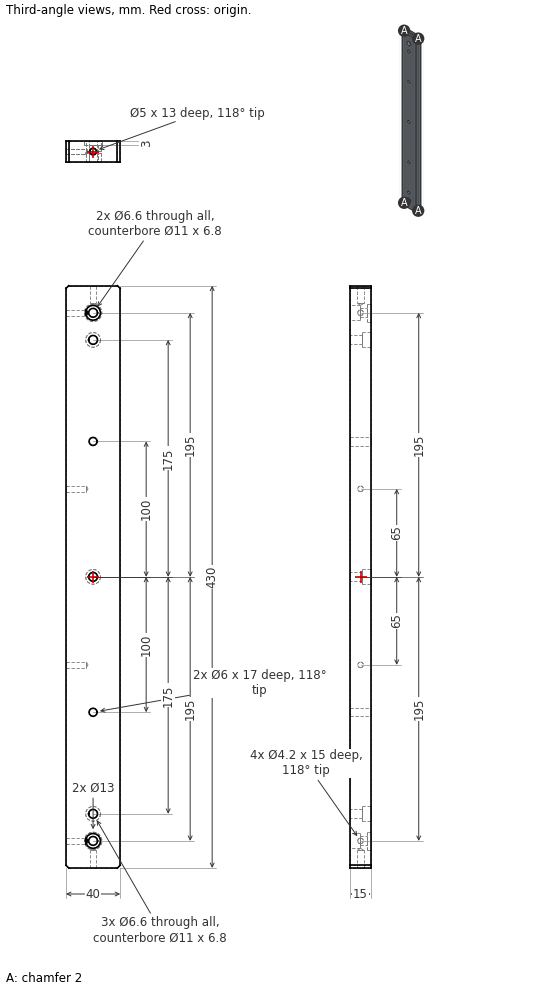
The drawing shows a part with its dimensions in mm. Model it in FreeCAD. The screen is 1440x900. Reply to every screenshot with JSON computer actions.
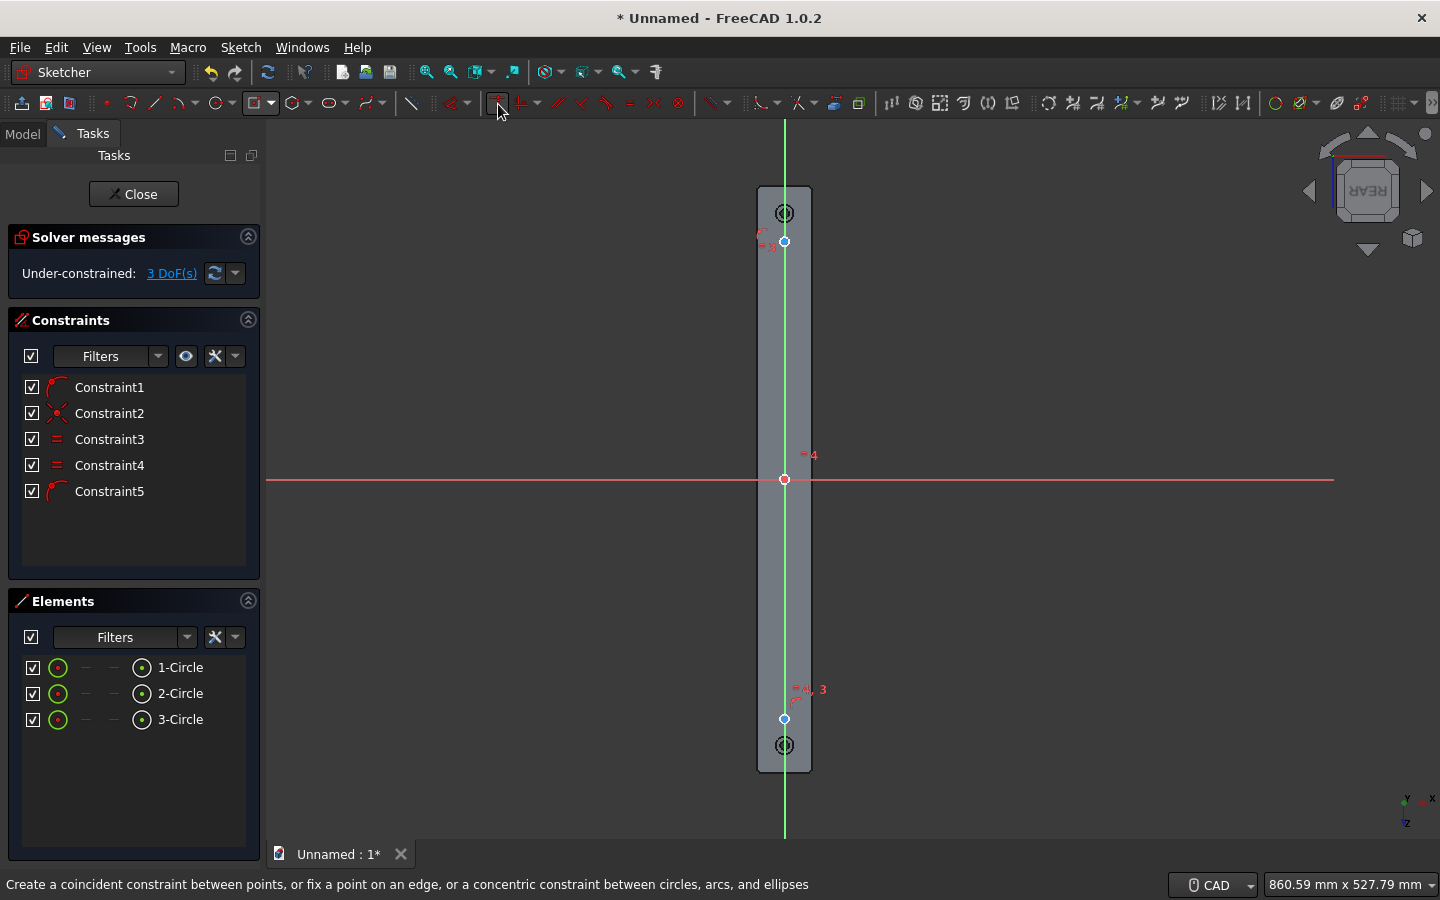
{"action": "key", "text": "d"}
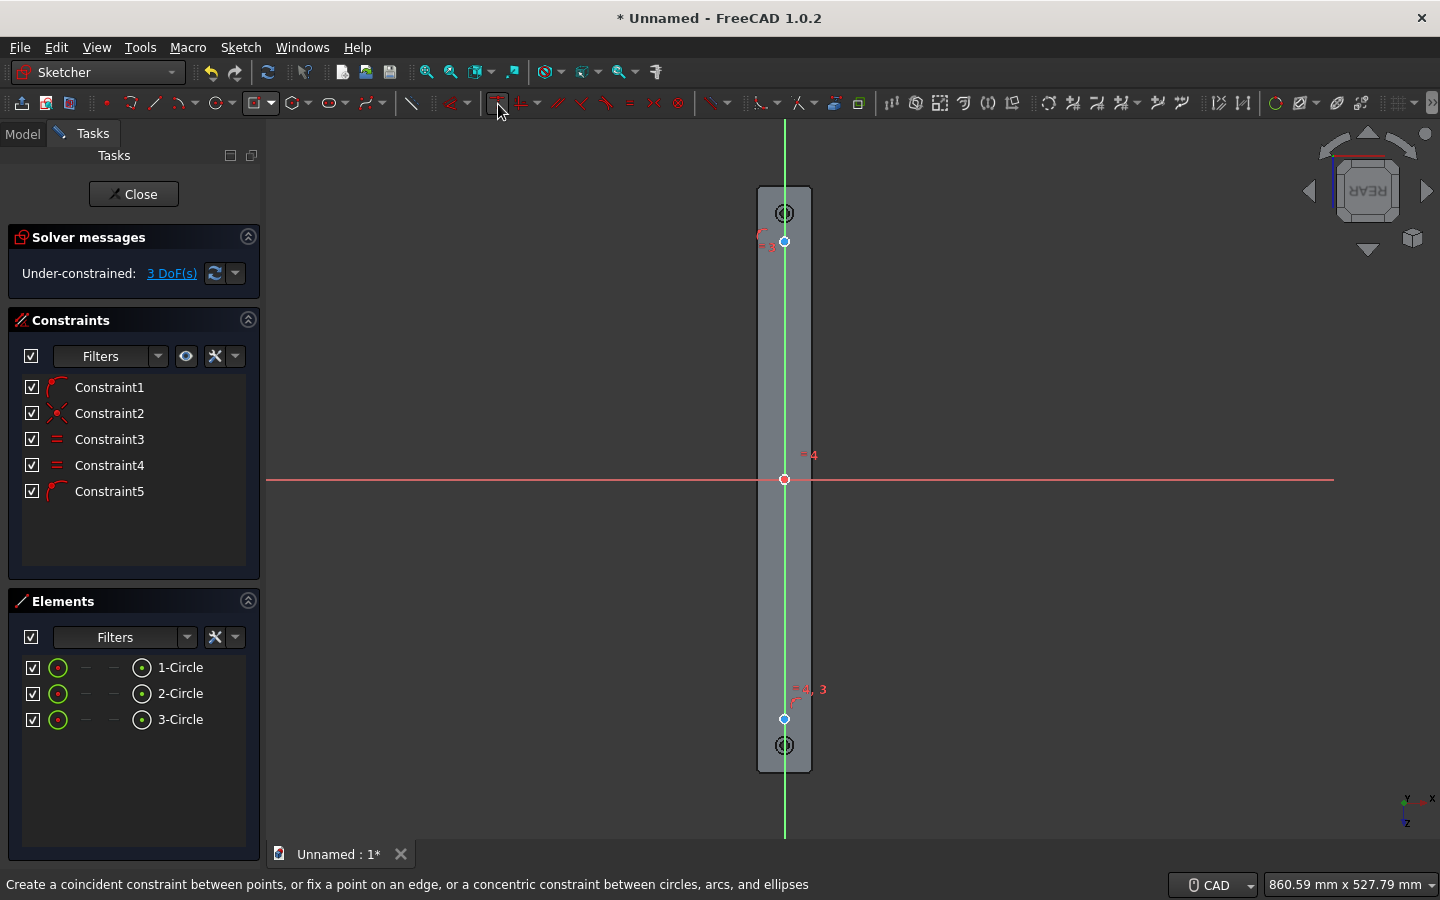
{"action": "scroll", "coordinate": [785, 237], "scroll_direction": "up", "scroll_amount": 8}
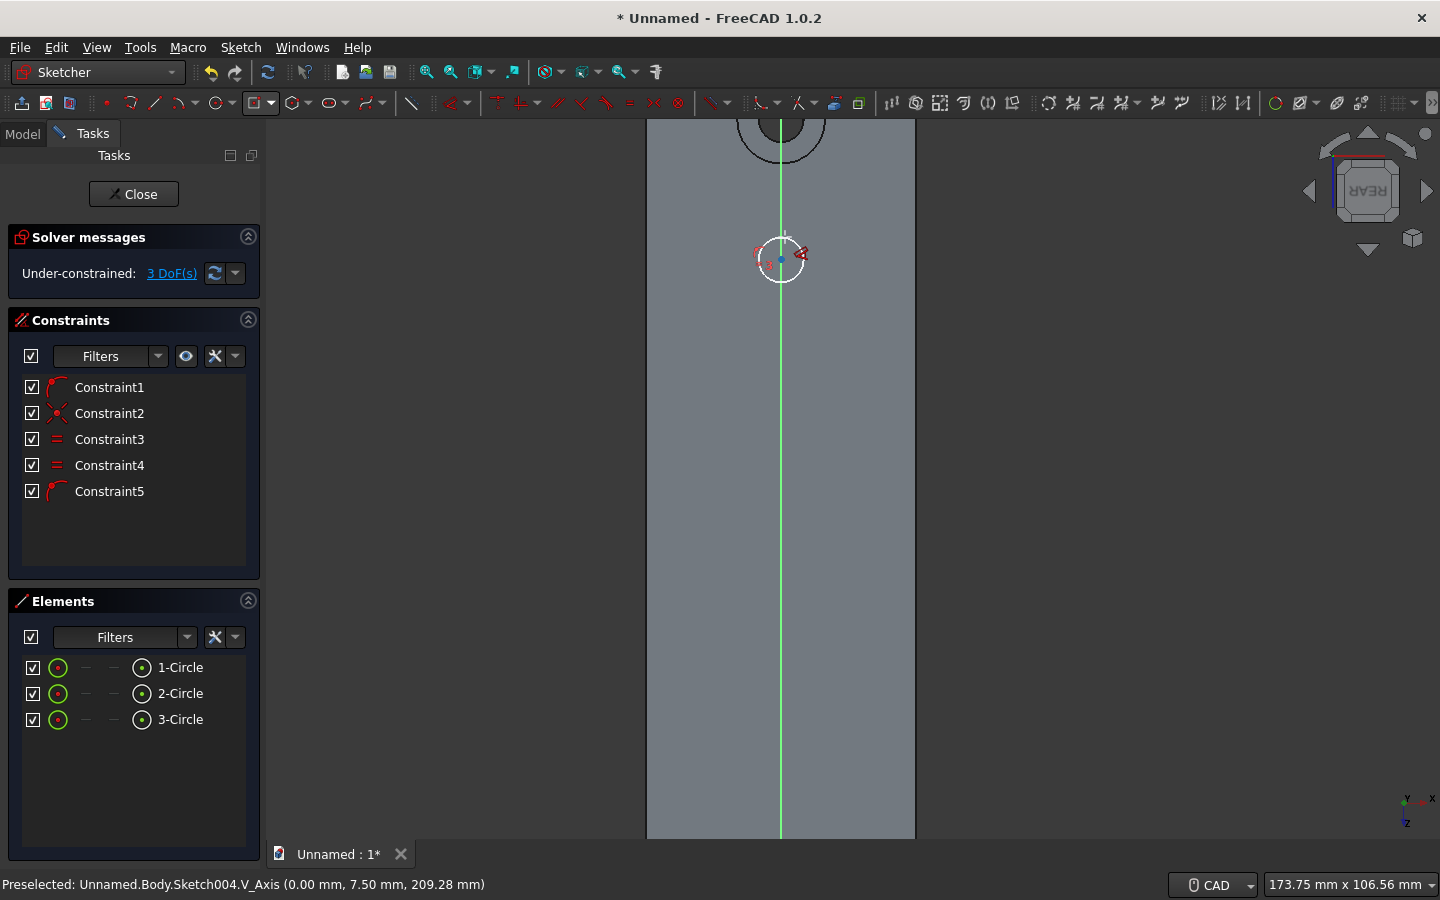
{"action": "left_click", "coordinate": [782, 238]}
{"action": "left_click", "coordinate": [809, 214]}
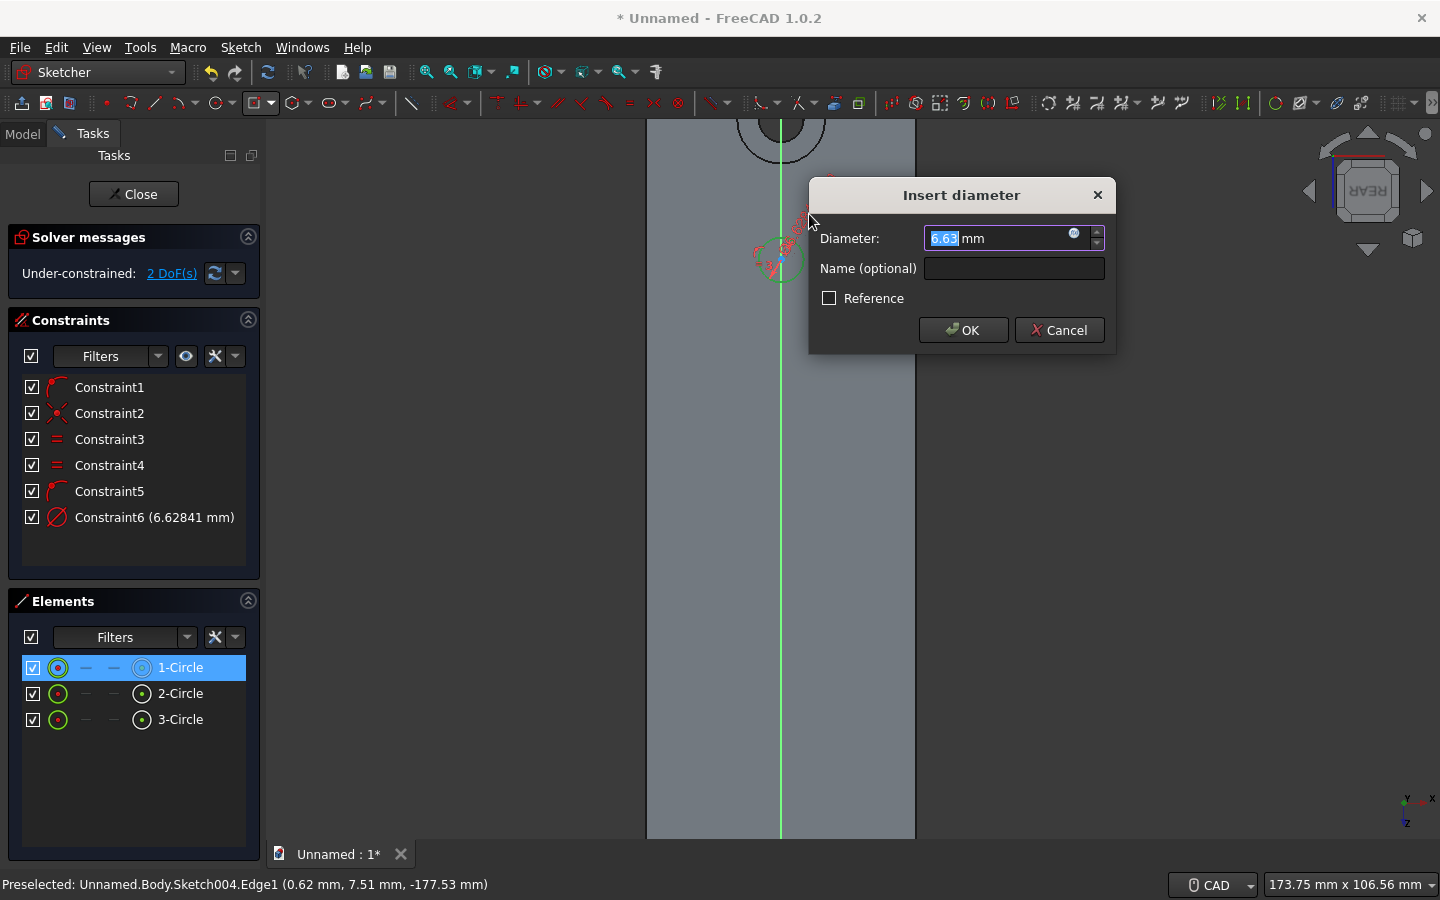
{"action": "type", "text": "6.6"}
{"action": "key", "text": "Return"}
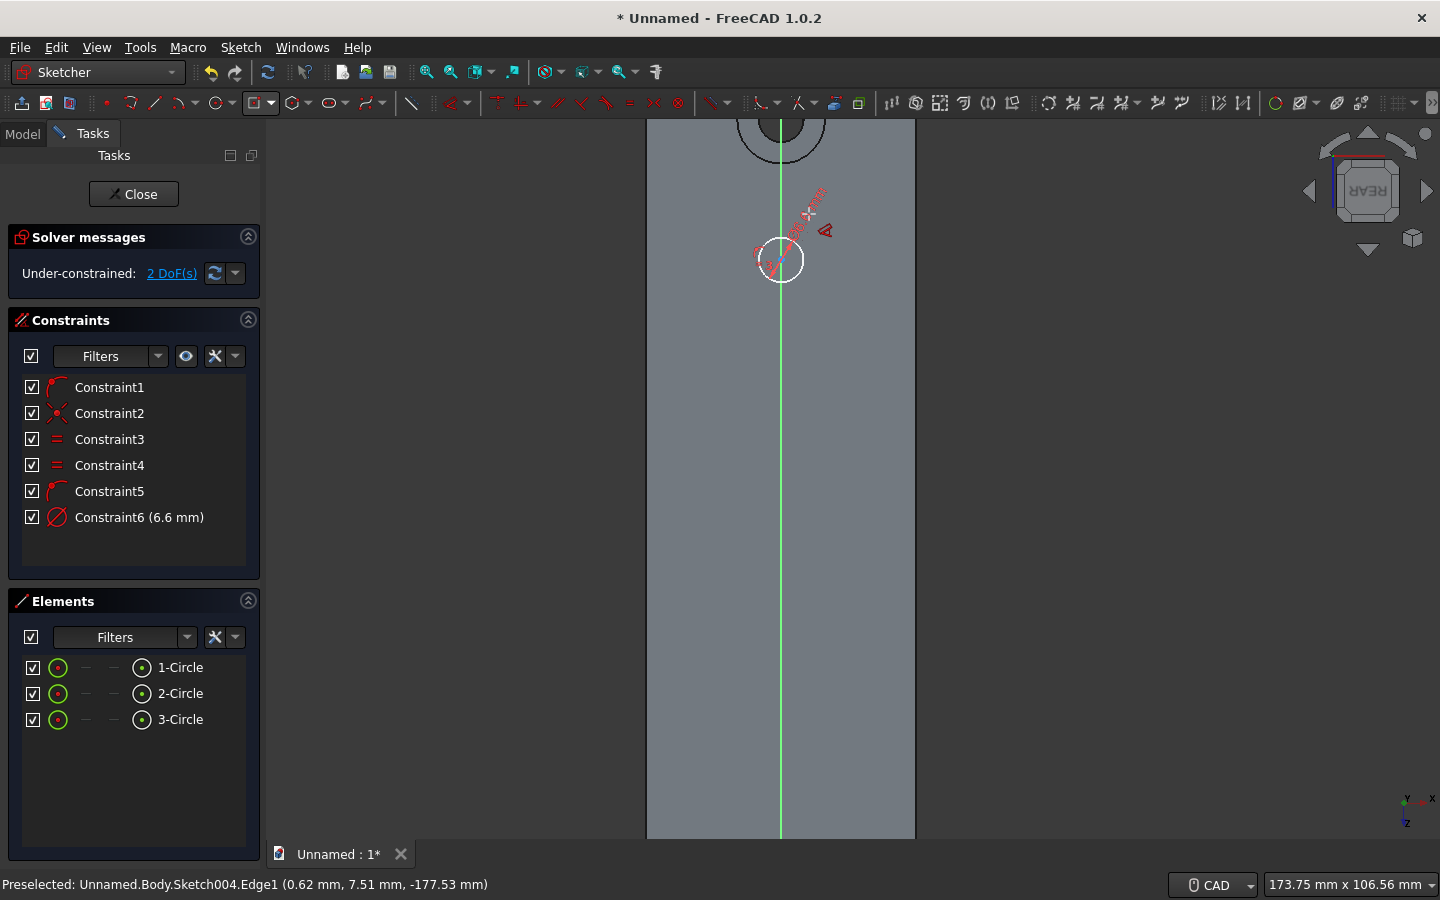
{"action": "scroll", "coordinate": [785, 237], "scroll_direction": "down", "scroll_amount": 8}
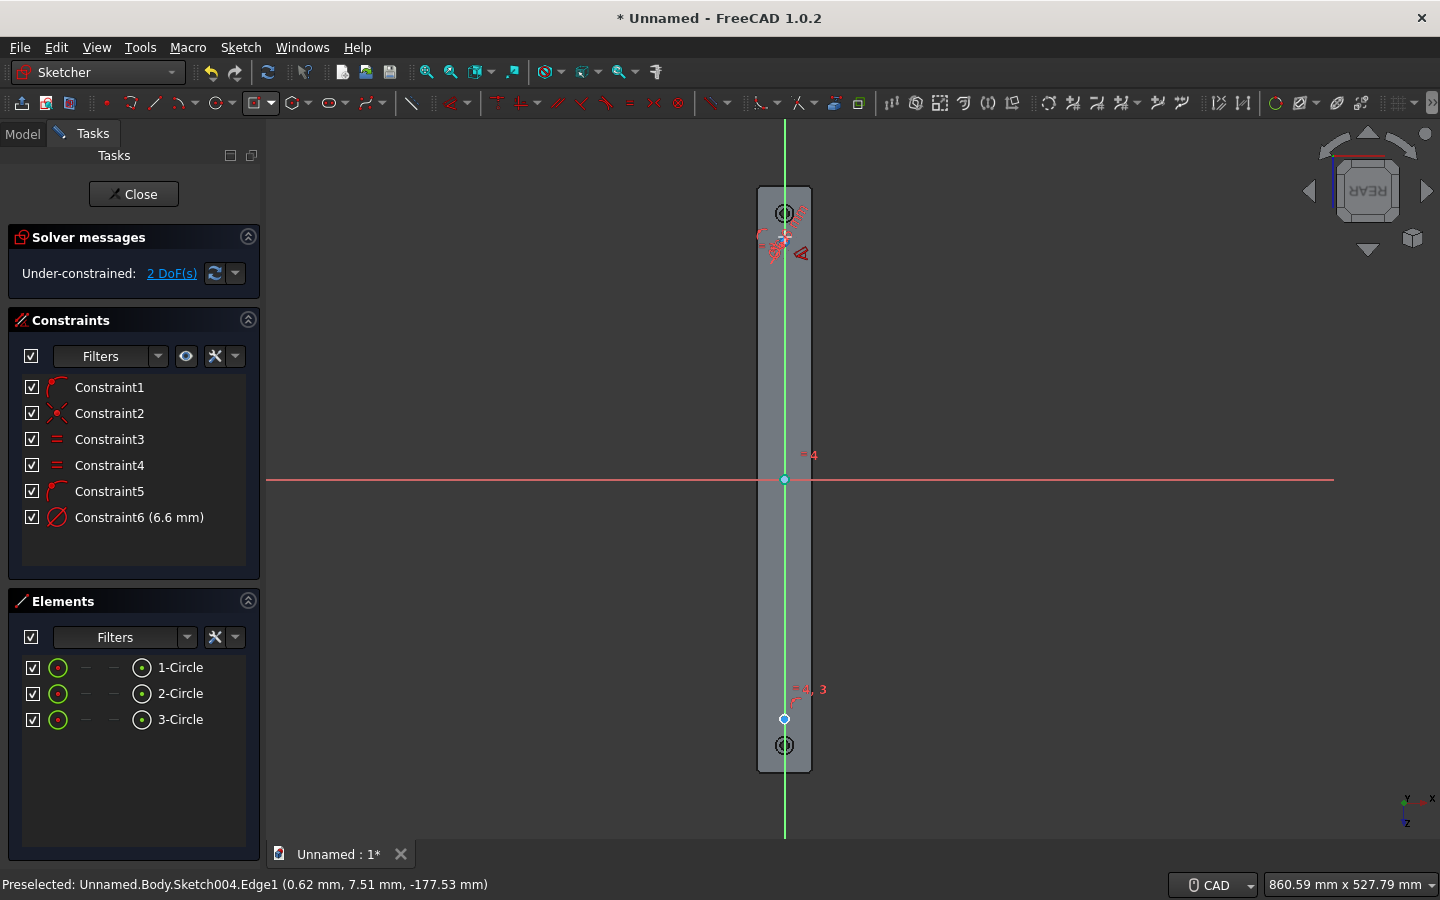
{"action": "left_click", "coordinate": [785, 242]}
{"action": "left_click", "coordinate": [819, 361]}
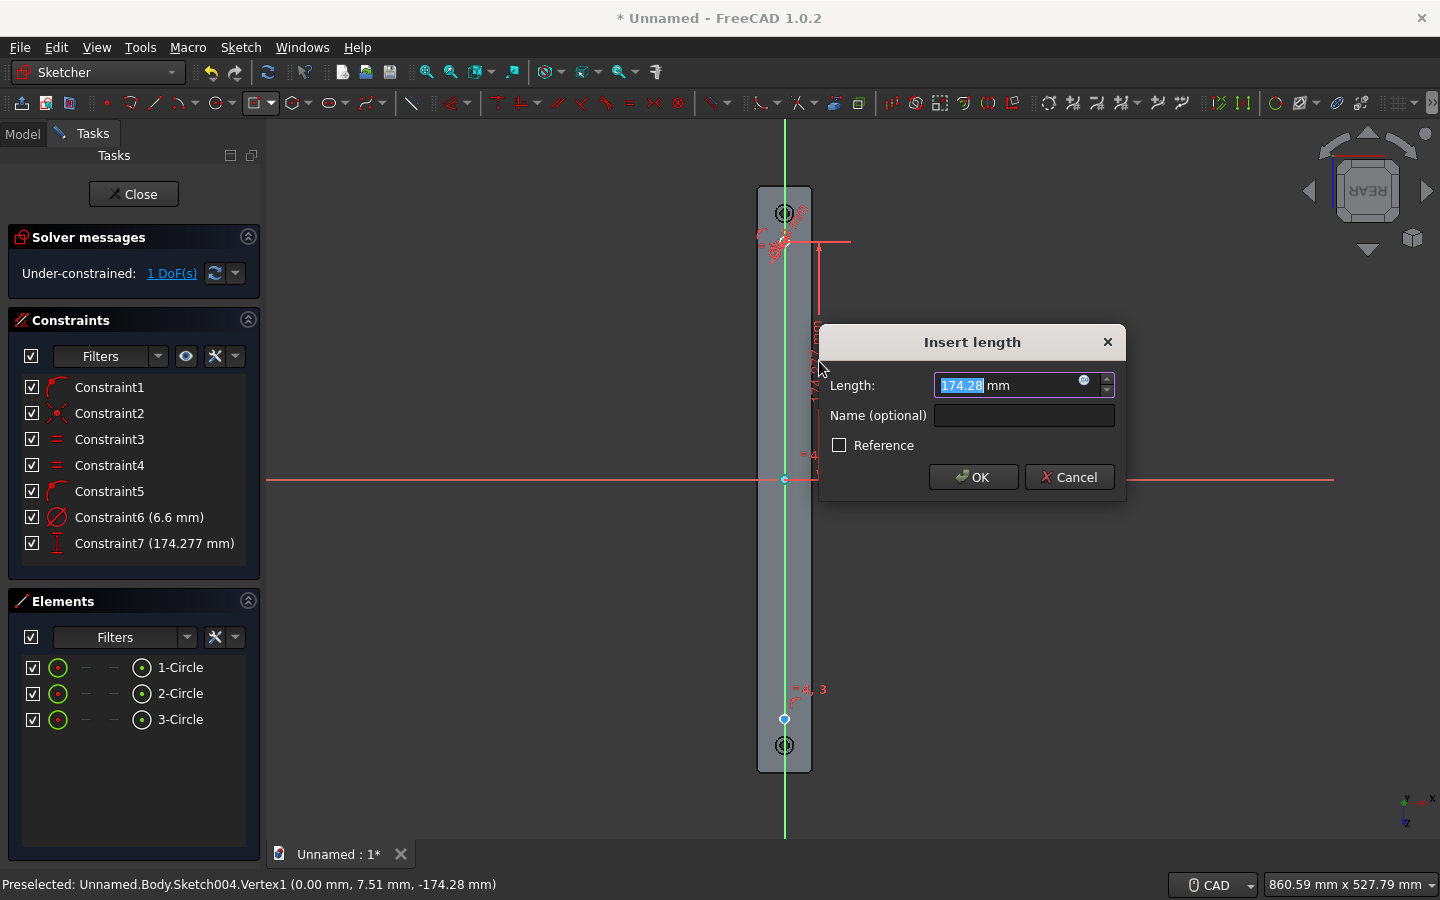
{"action": "type", "text": "175"}
{"action": "key", "text": "Return"}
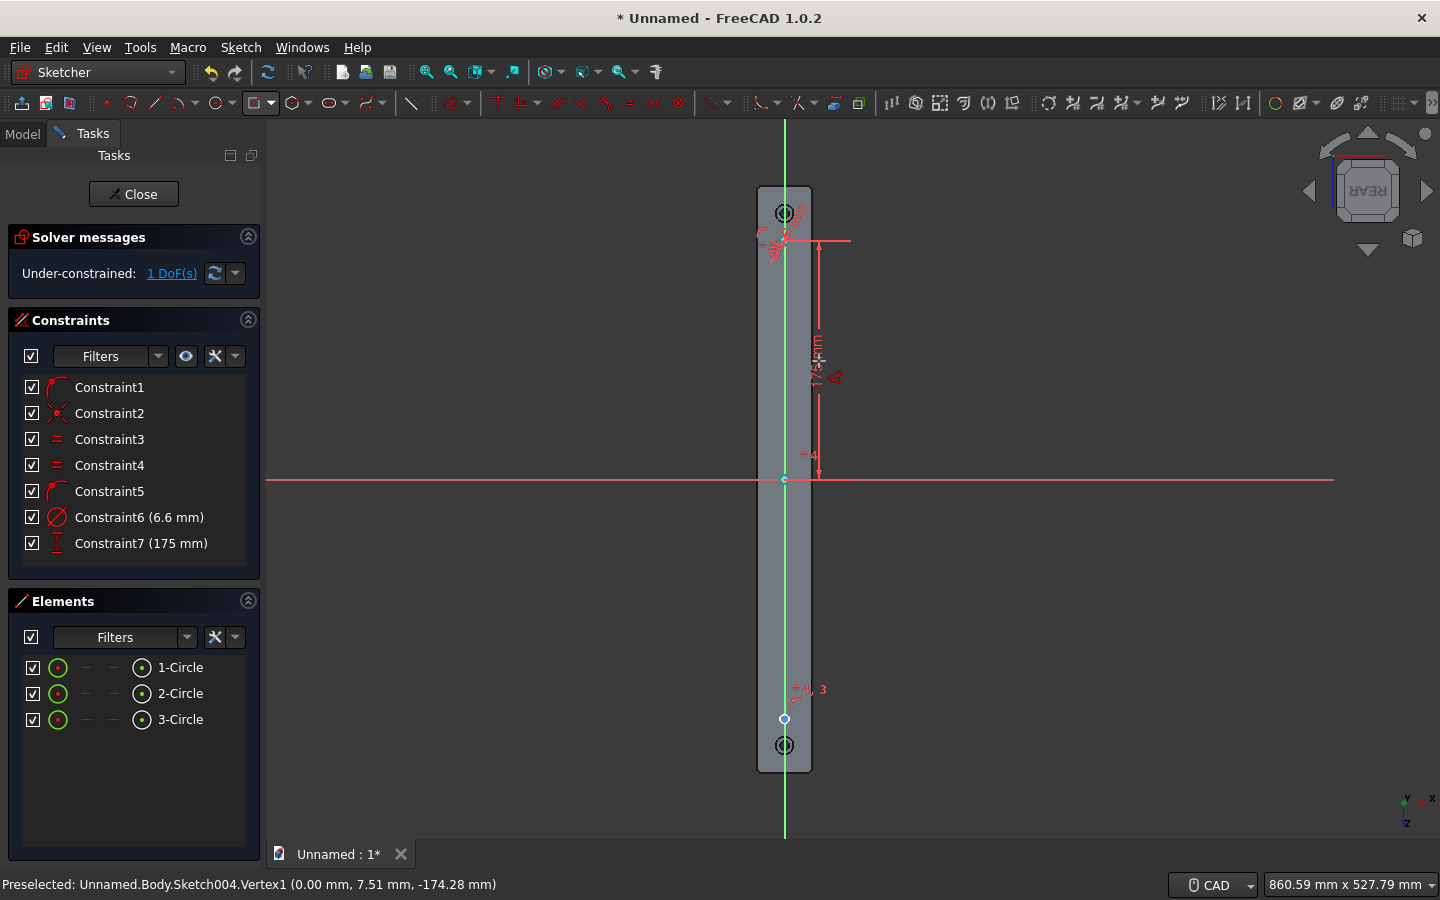
{"action": "left_click", "coordinate": [785, 719]}
{"action": "left_click", "coordinate": [819, 599]}